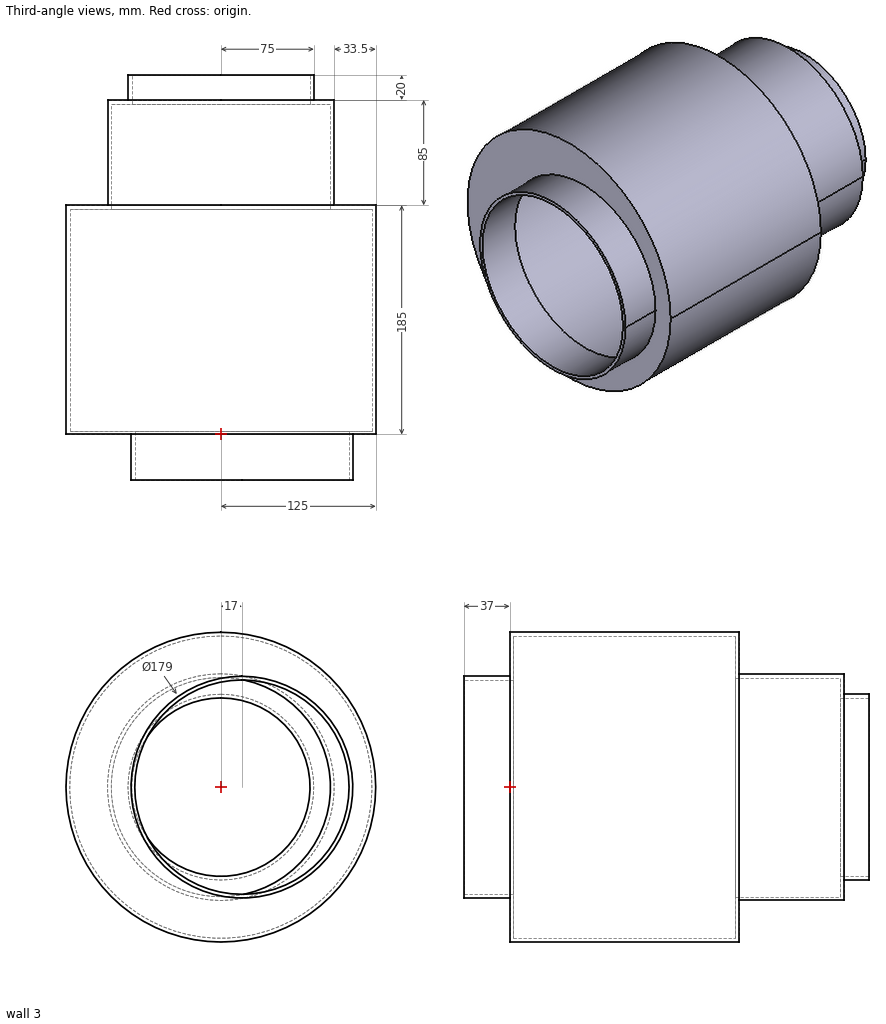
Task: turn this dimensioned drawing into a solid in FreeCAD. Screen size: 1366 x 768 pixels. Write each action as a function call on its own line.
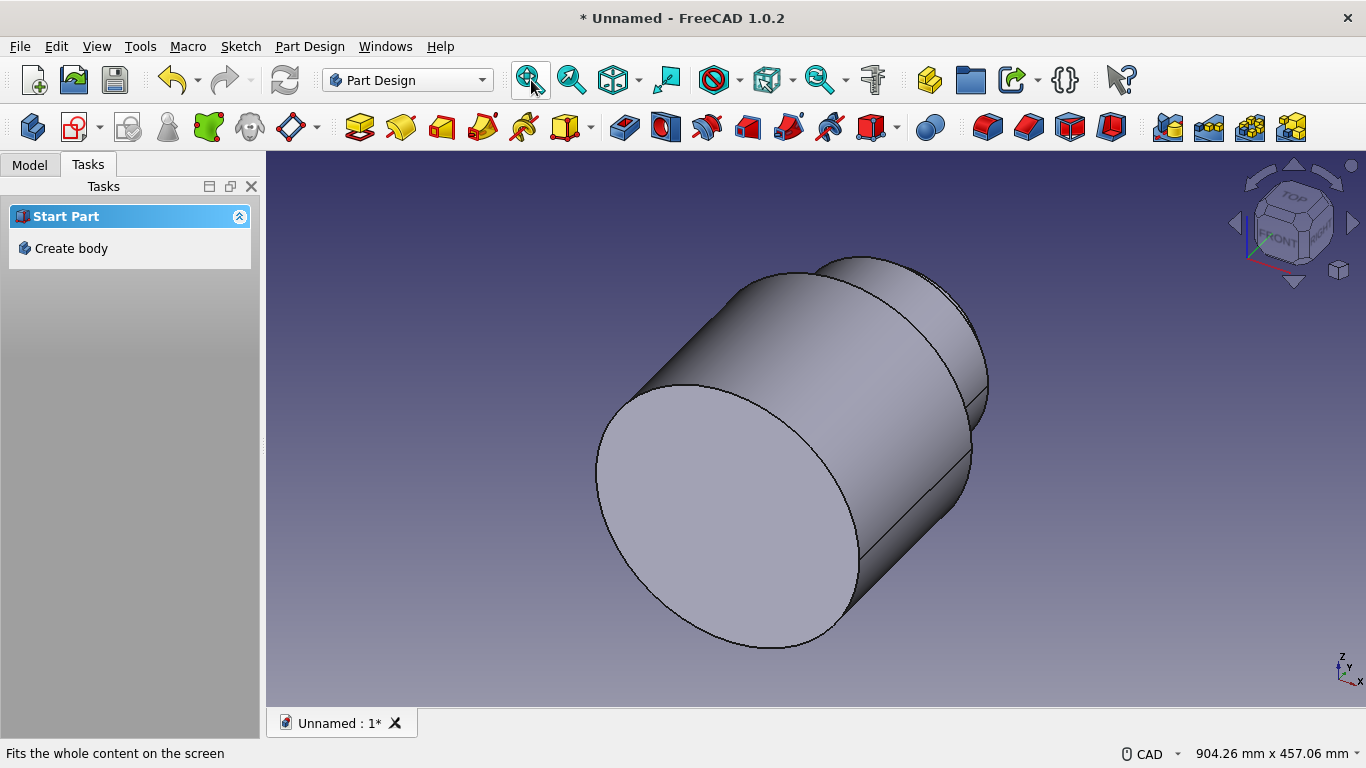
click(74, 128)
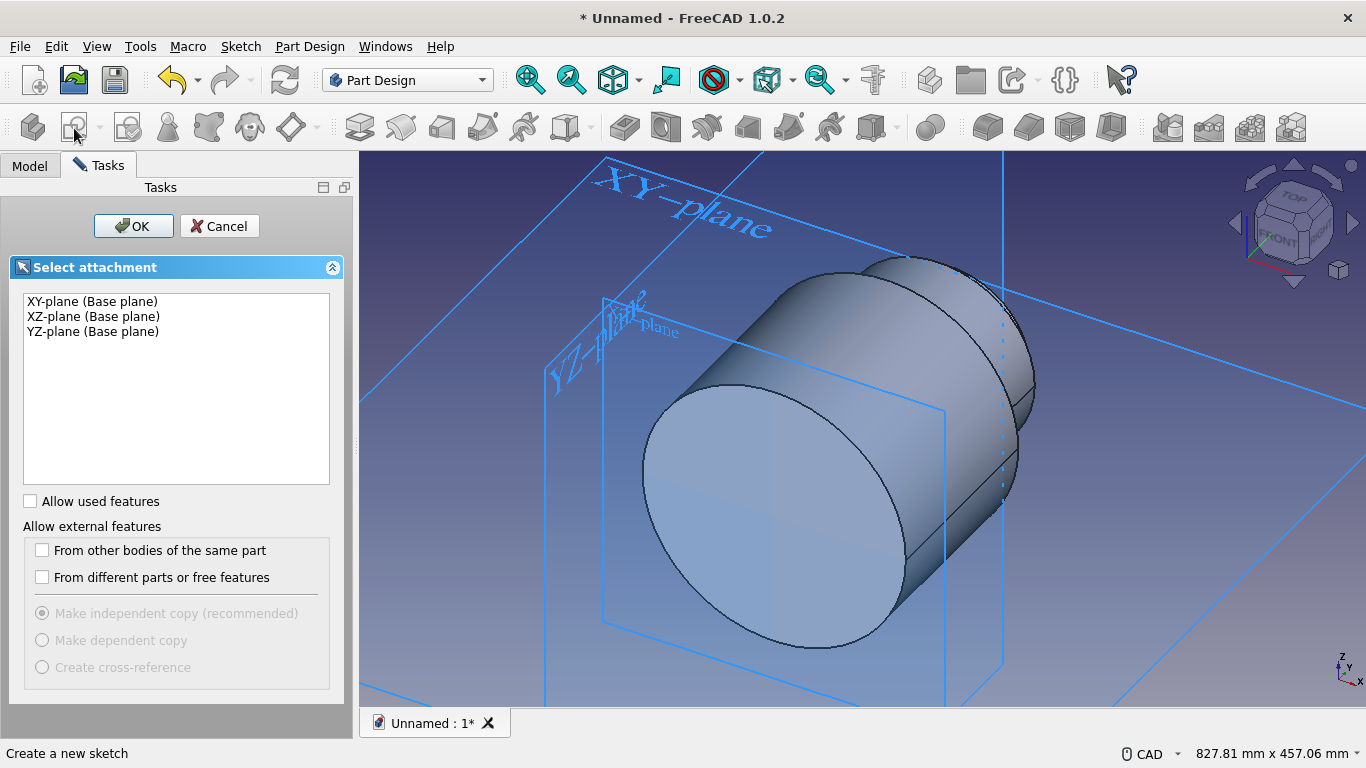
click(84, 316)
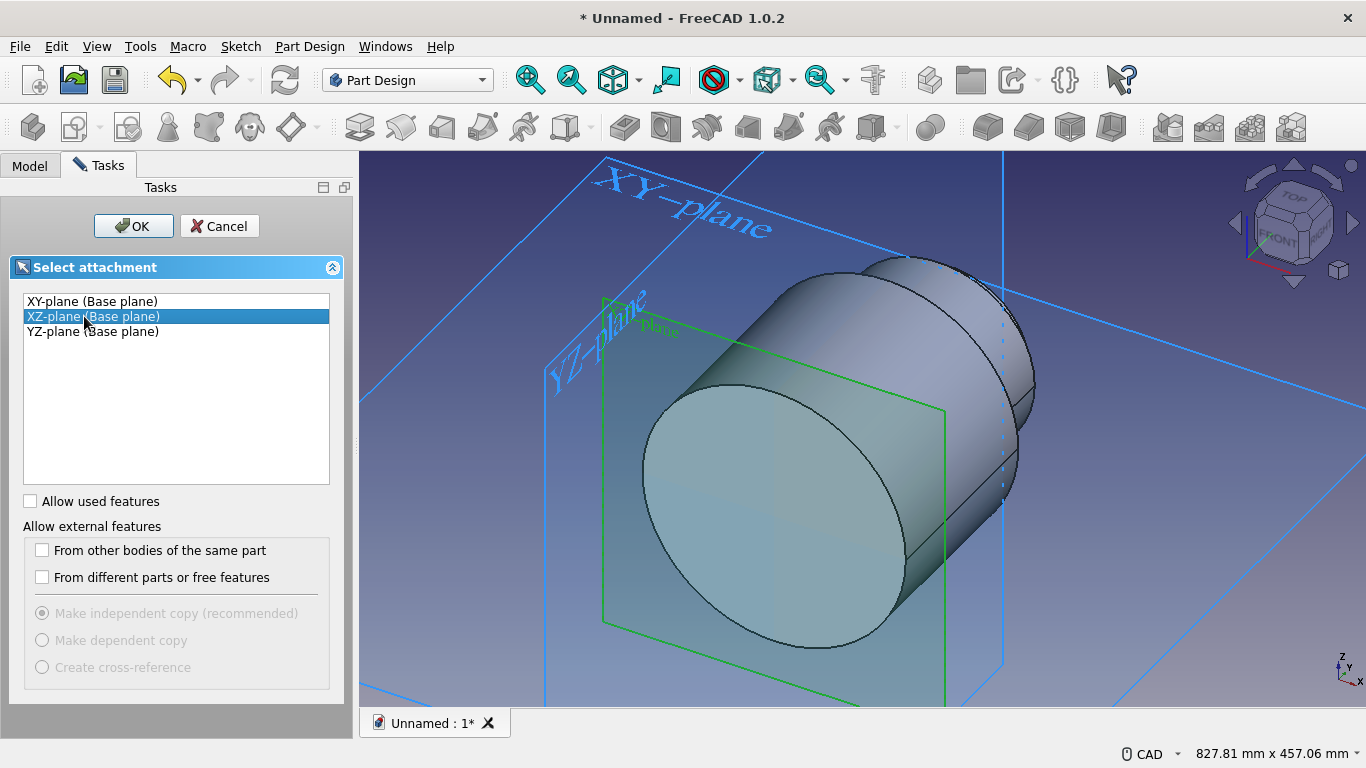
click(134, 226)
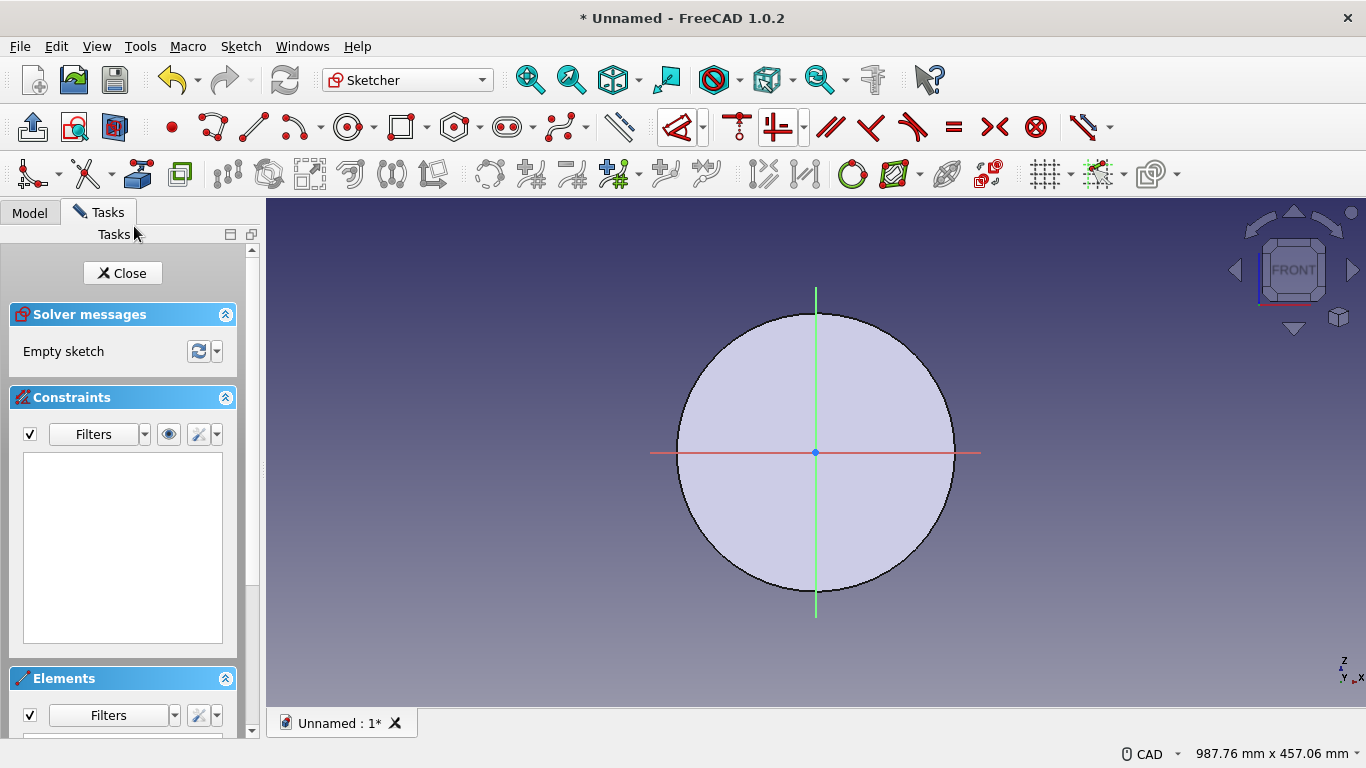
scroll(1012, 453, up, 2)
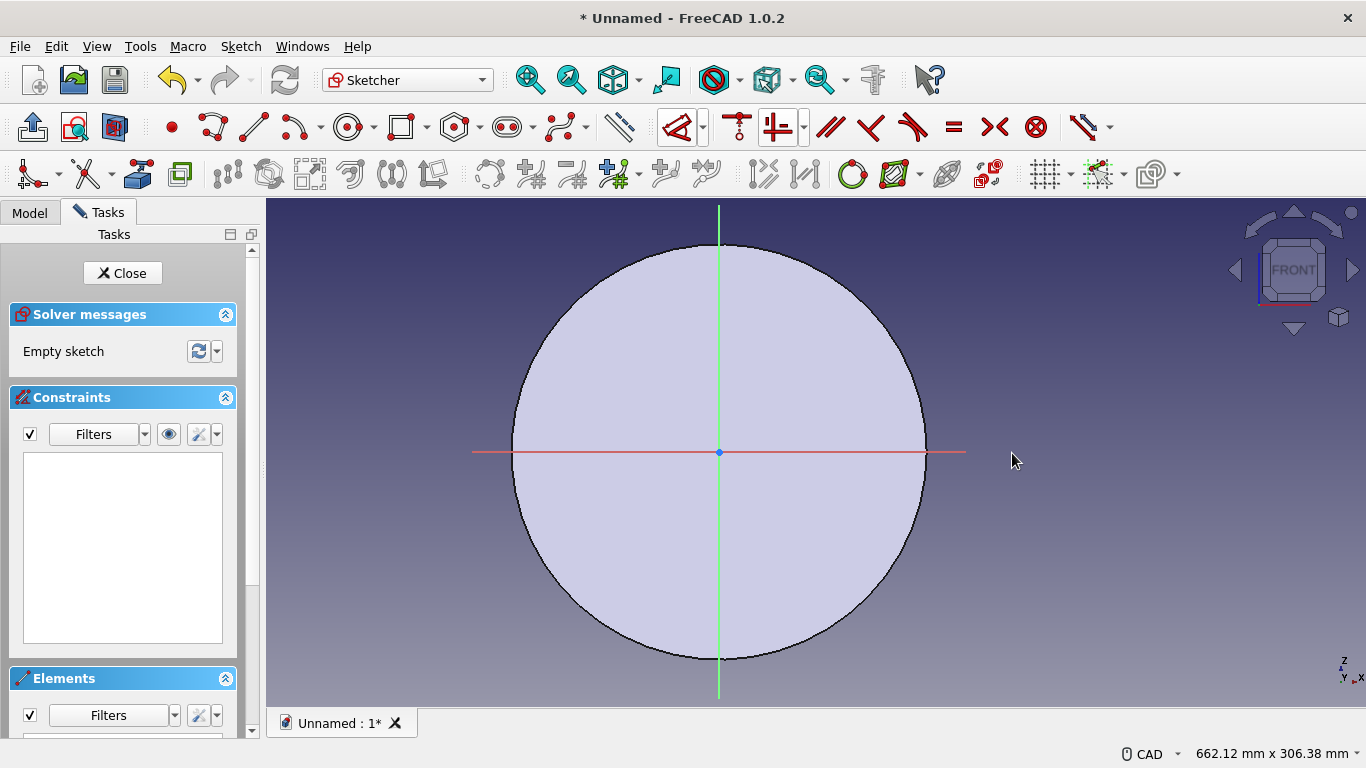
click(348, 128)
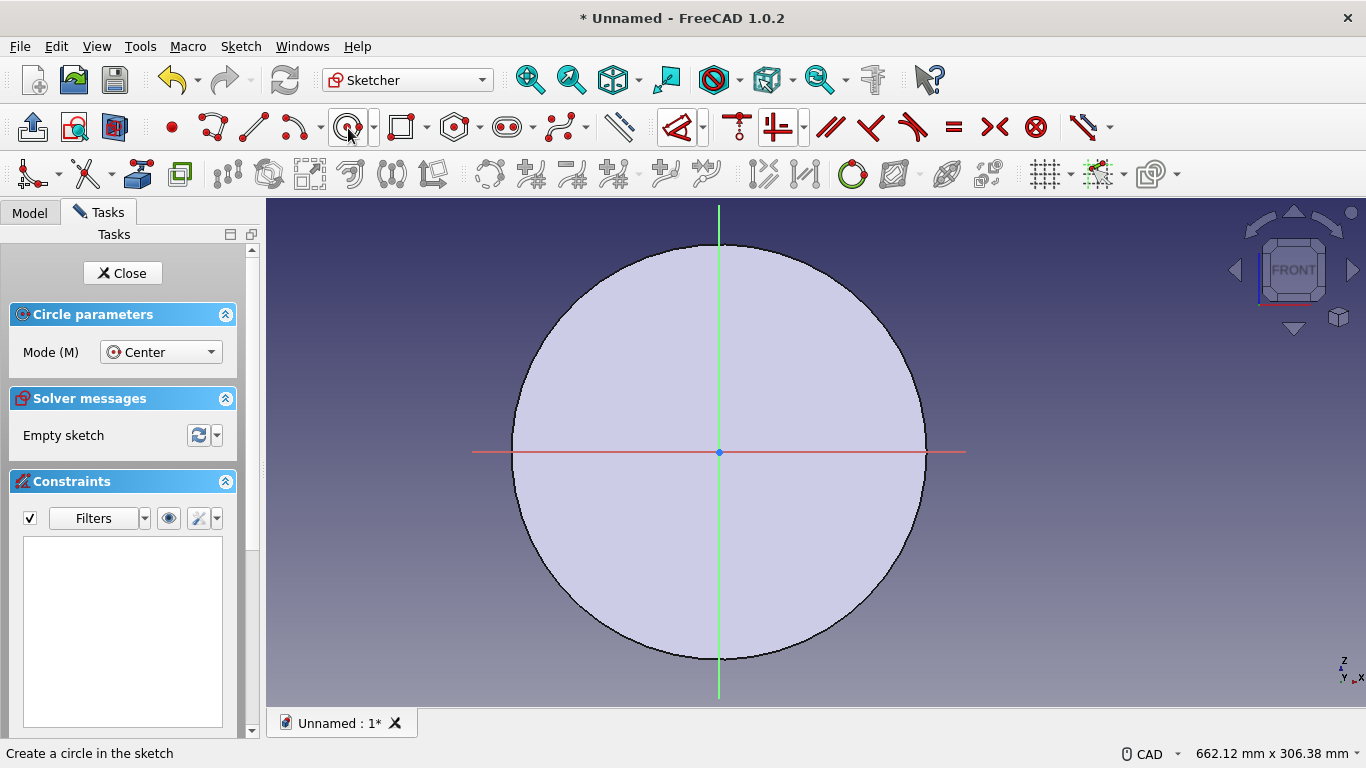
click(747, 452)
move(852, 347)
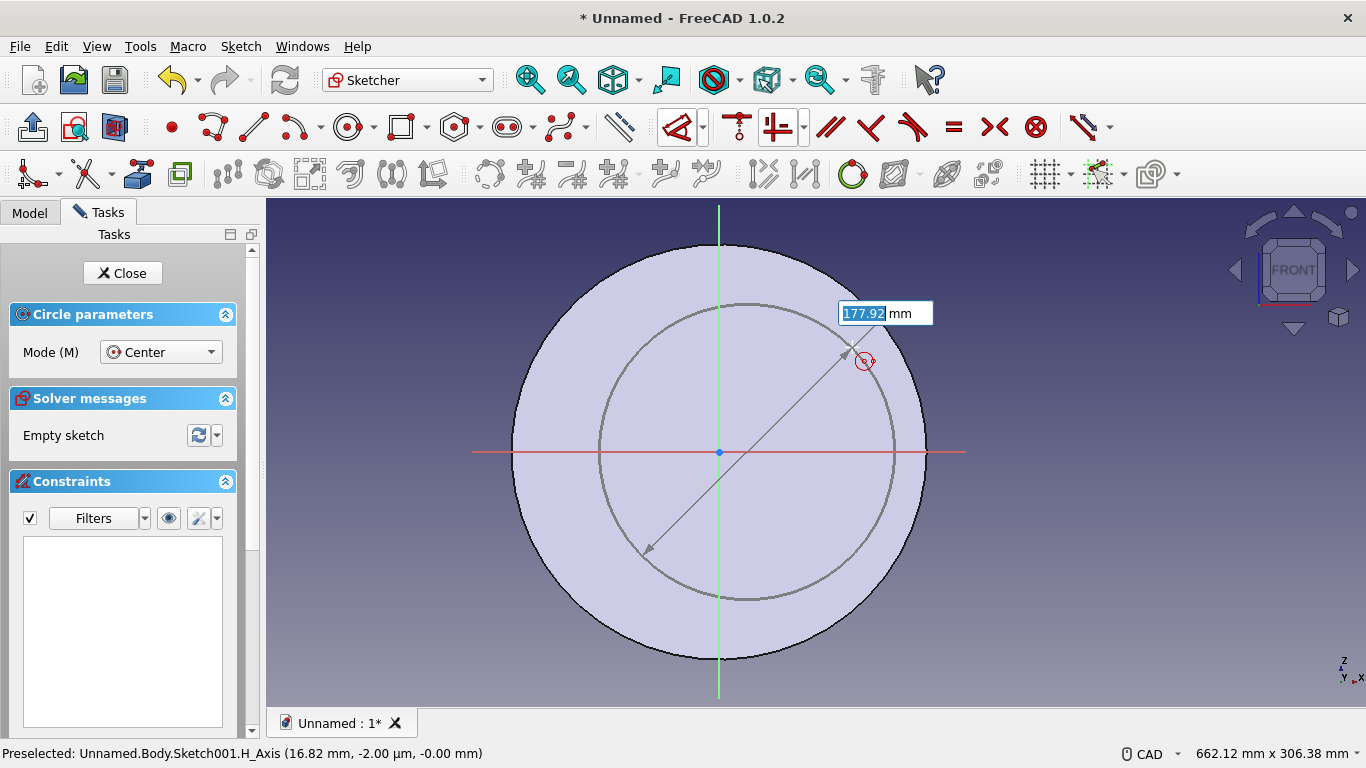
text(179)
key(Return)
key(Escape)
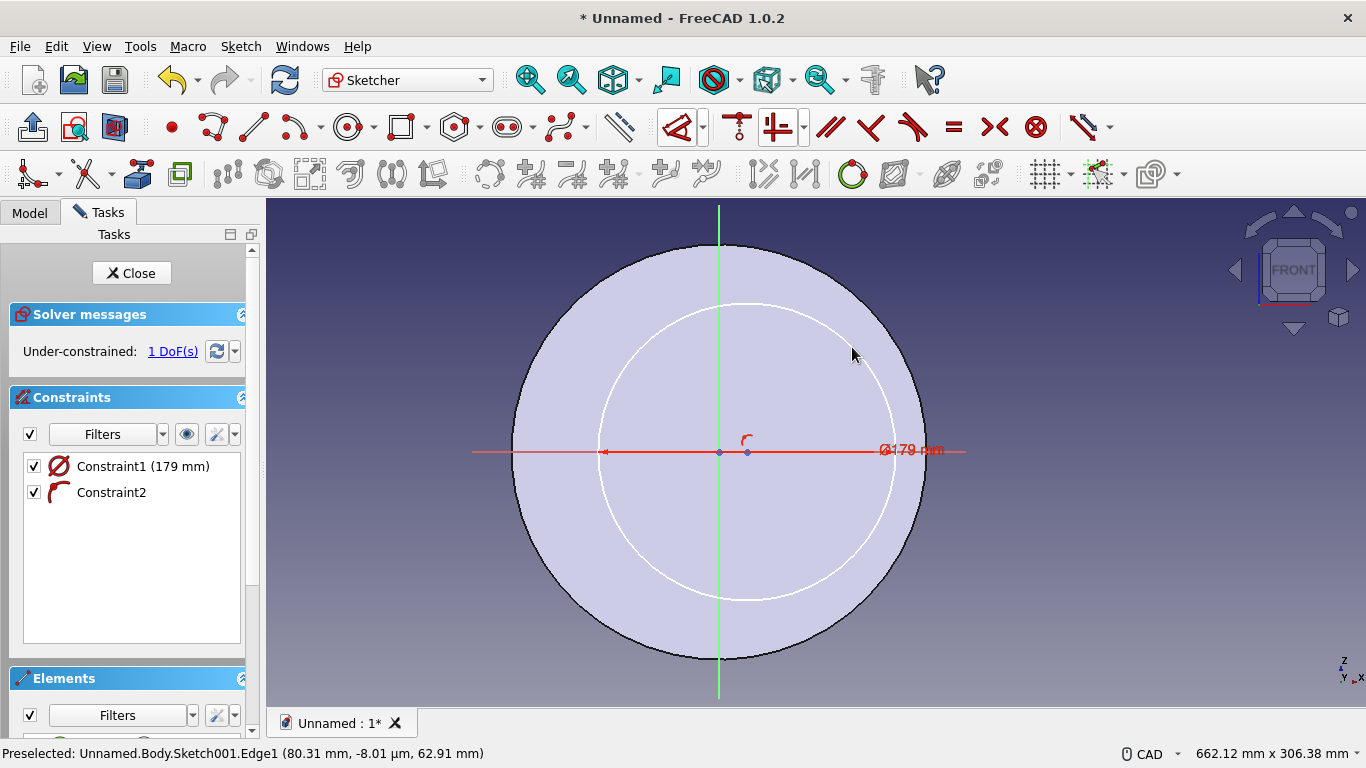
scroll(747, 452, up, 2)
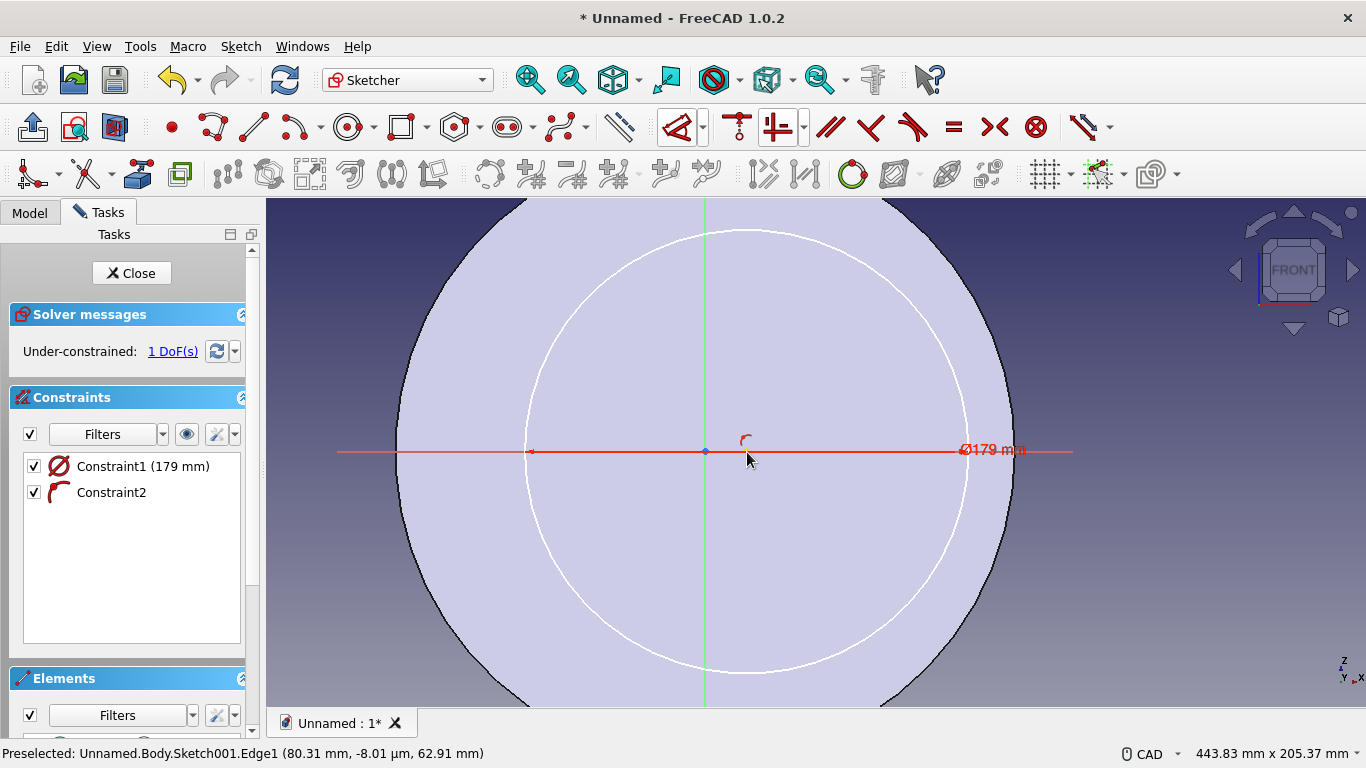
click(747, 452)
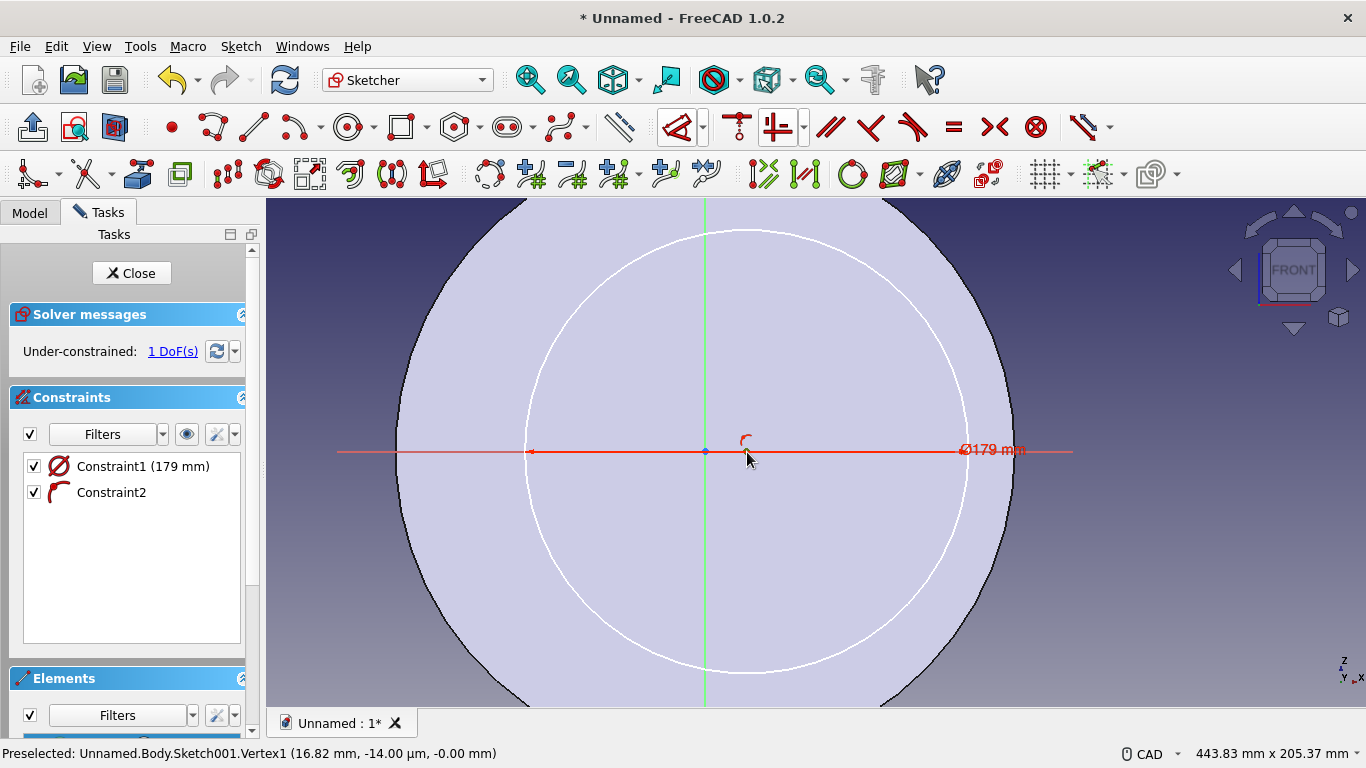
click(702, 128)